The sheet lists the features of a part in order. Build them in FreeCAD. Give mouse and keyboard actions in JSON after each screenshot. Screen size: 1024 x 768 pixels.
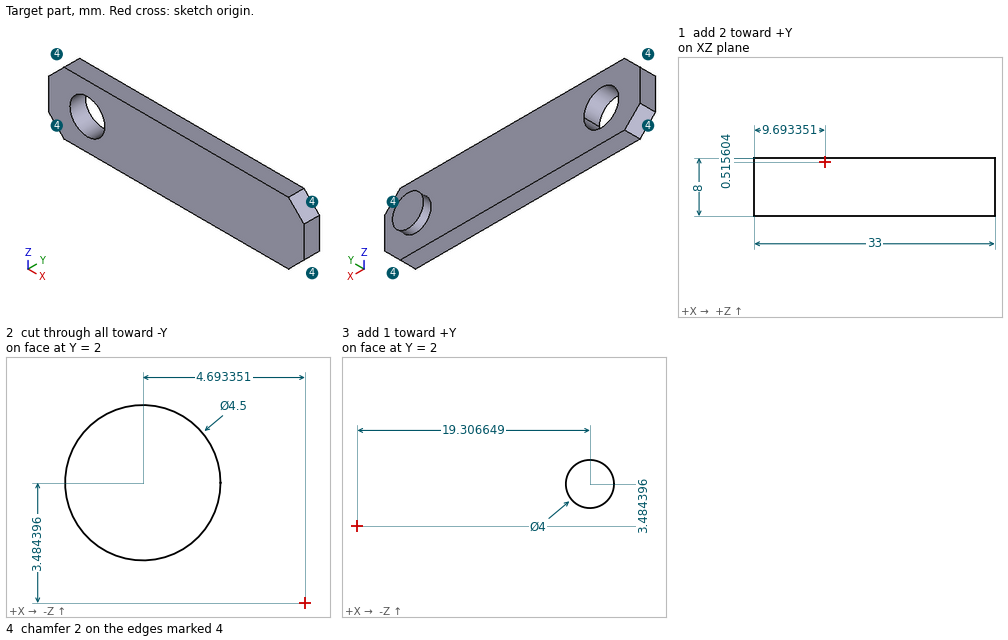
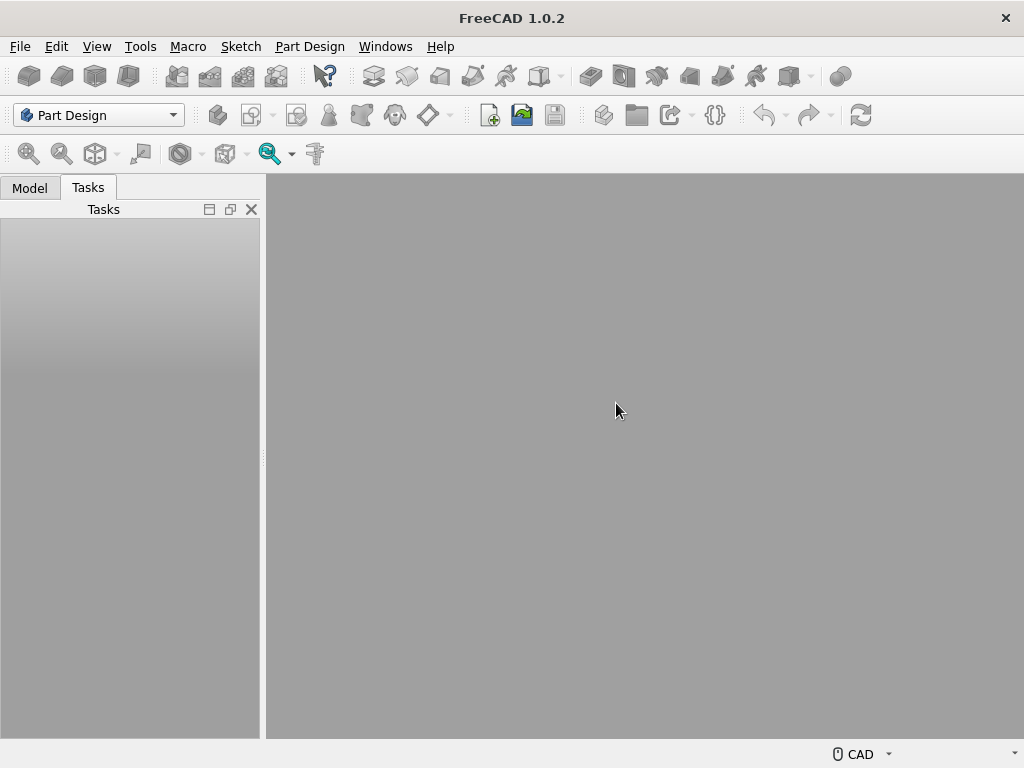
{"action": "key", "text": "ctrl+n"}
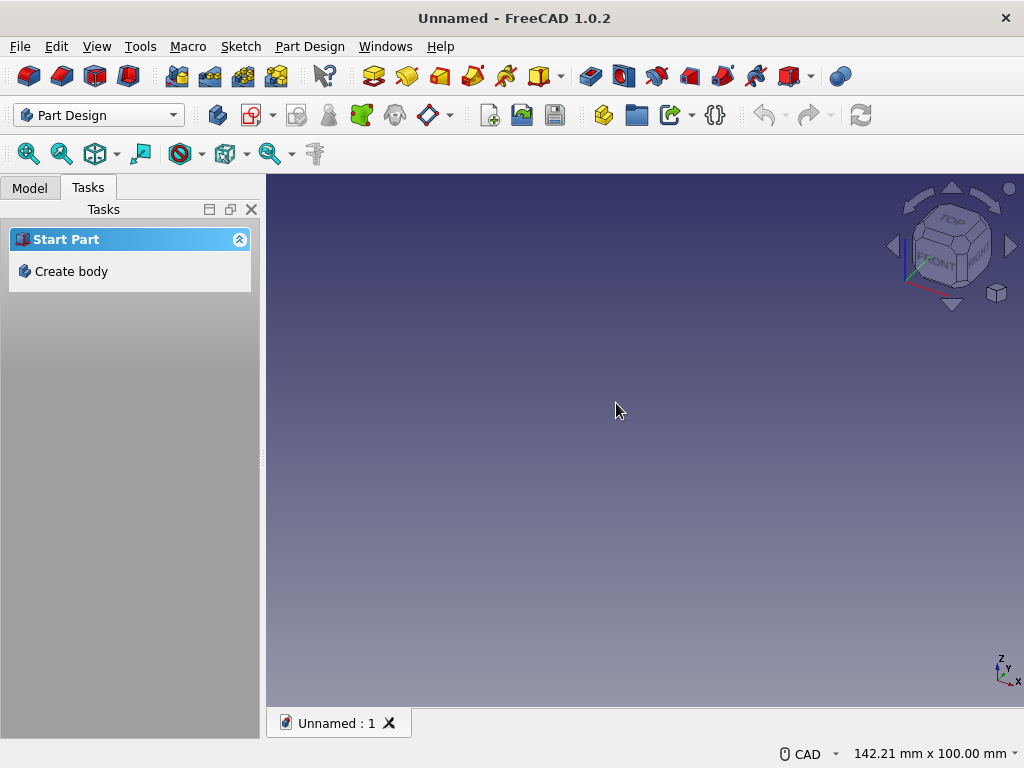
{"action": "left_click", "coordinate": [250, 116]}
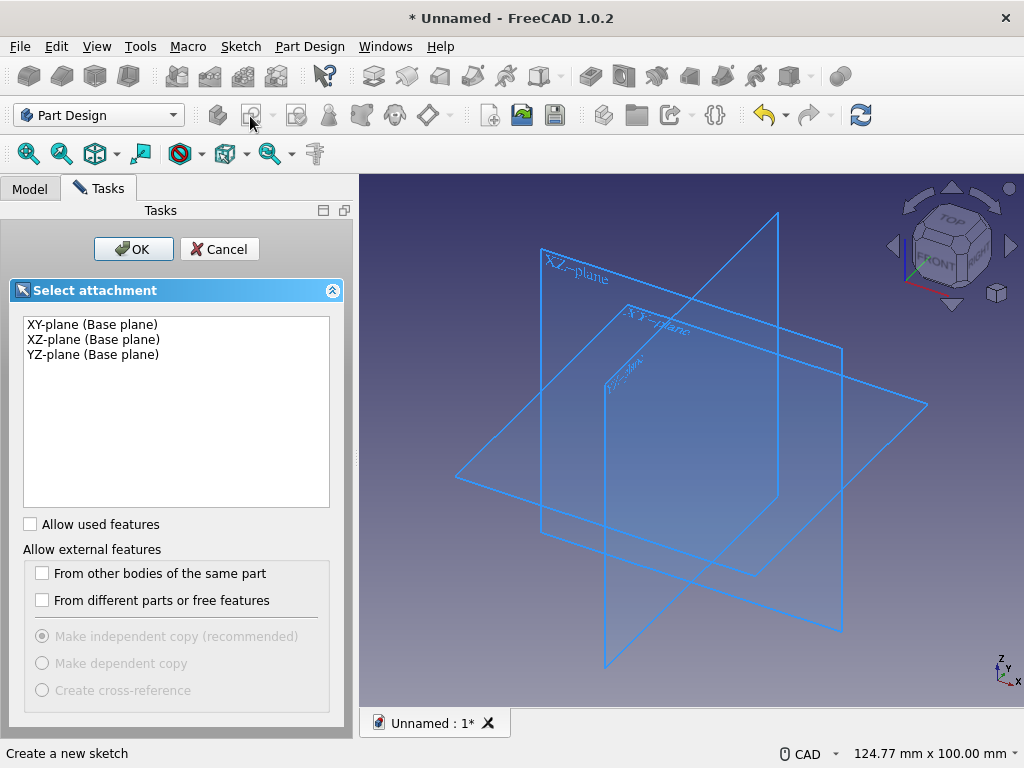
{"action": "left_click", "coordinate": [84, 340]}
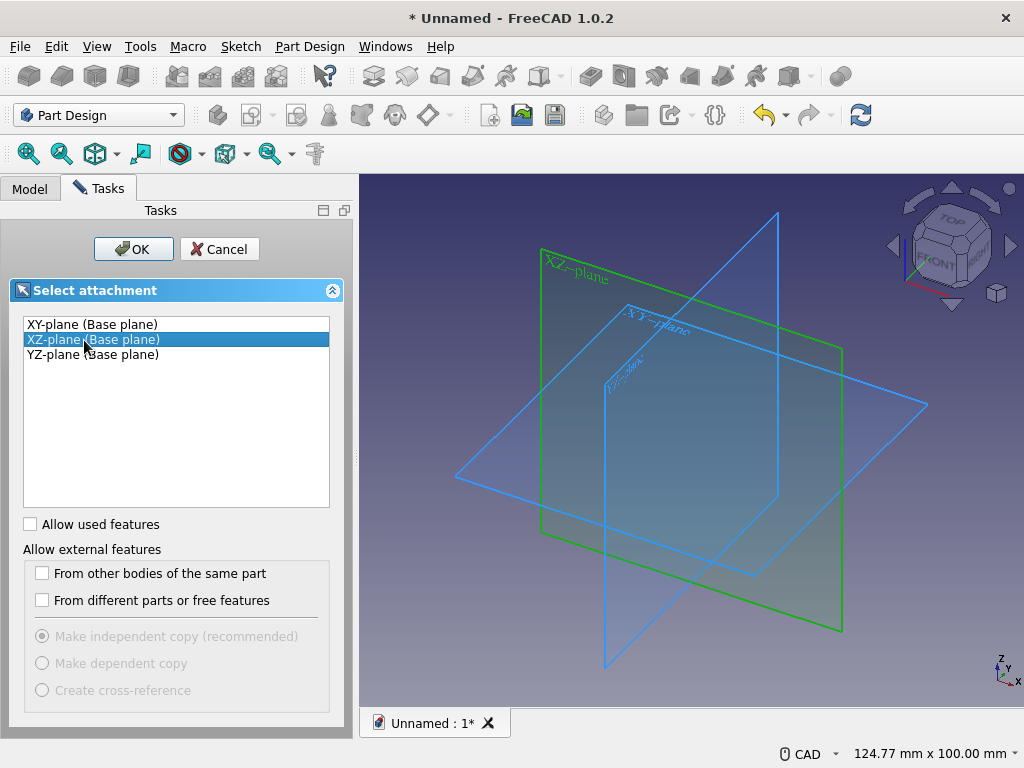
{"action": "left_click", "coordinate": [134, 249]}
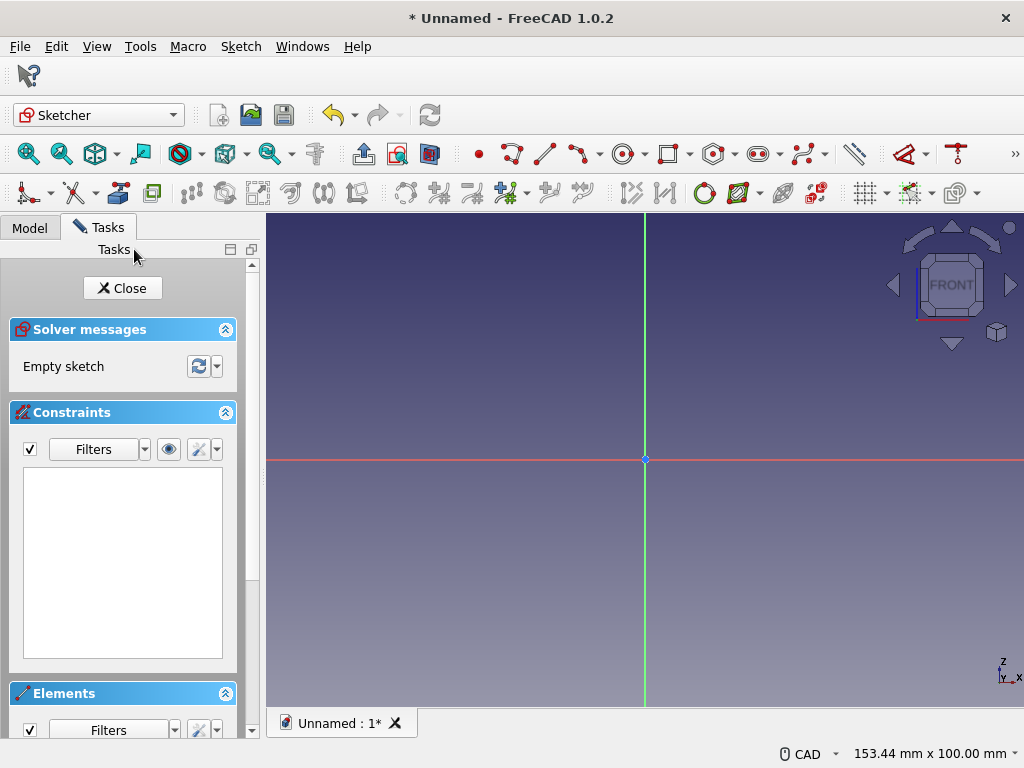
{"action": "scroll", "coordinate": [762, 491], "scroll_direction": "up", "scroll_amount": 4}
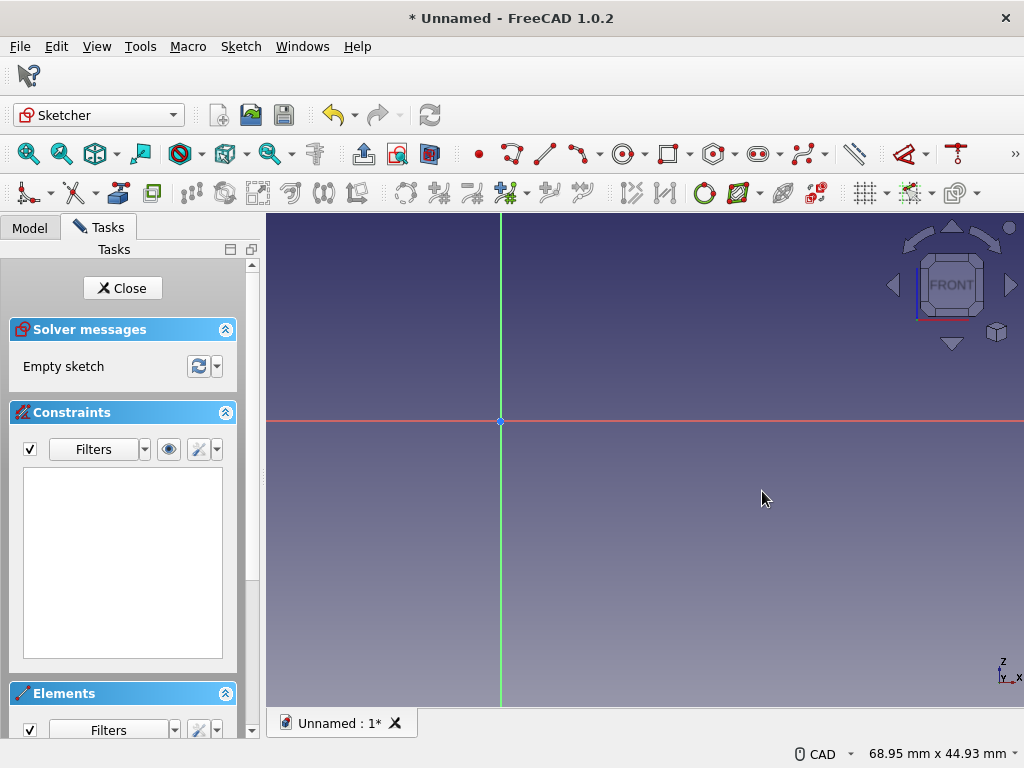
{"action": "left_click", "coordinate": [668, 154]}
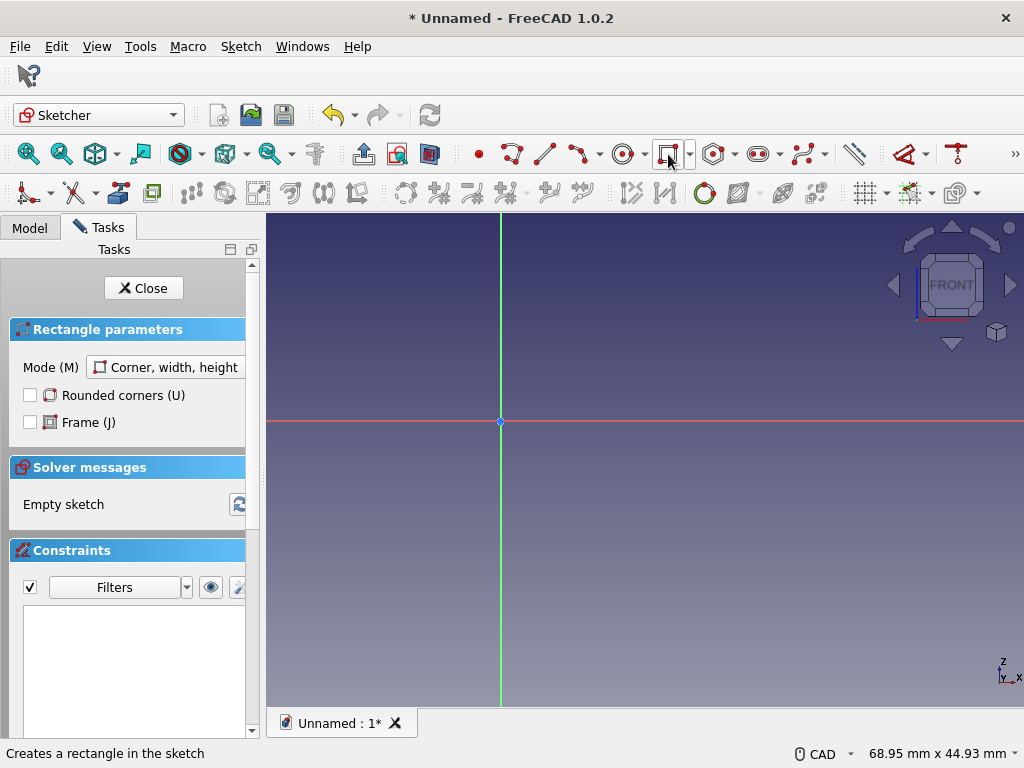
{"action": "scroll", "coordinate": [394, 416], "scroll_direction": "up", "scroll_amount": 6}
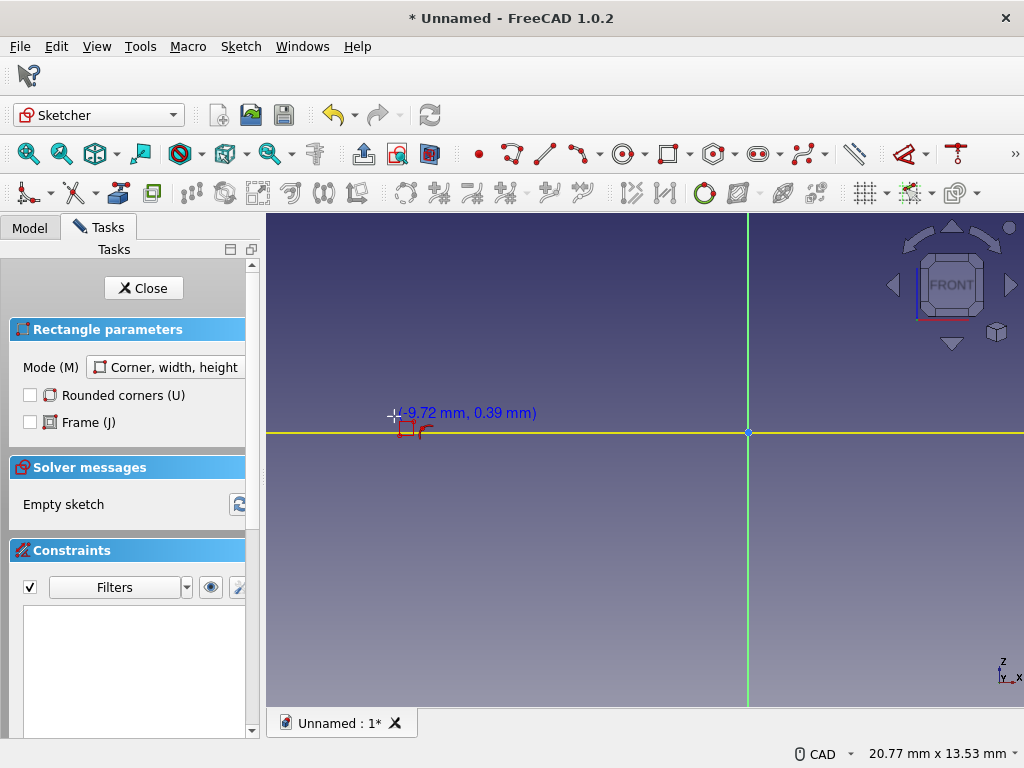
{"action": "left_click", "coordinate": [394, 414]}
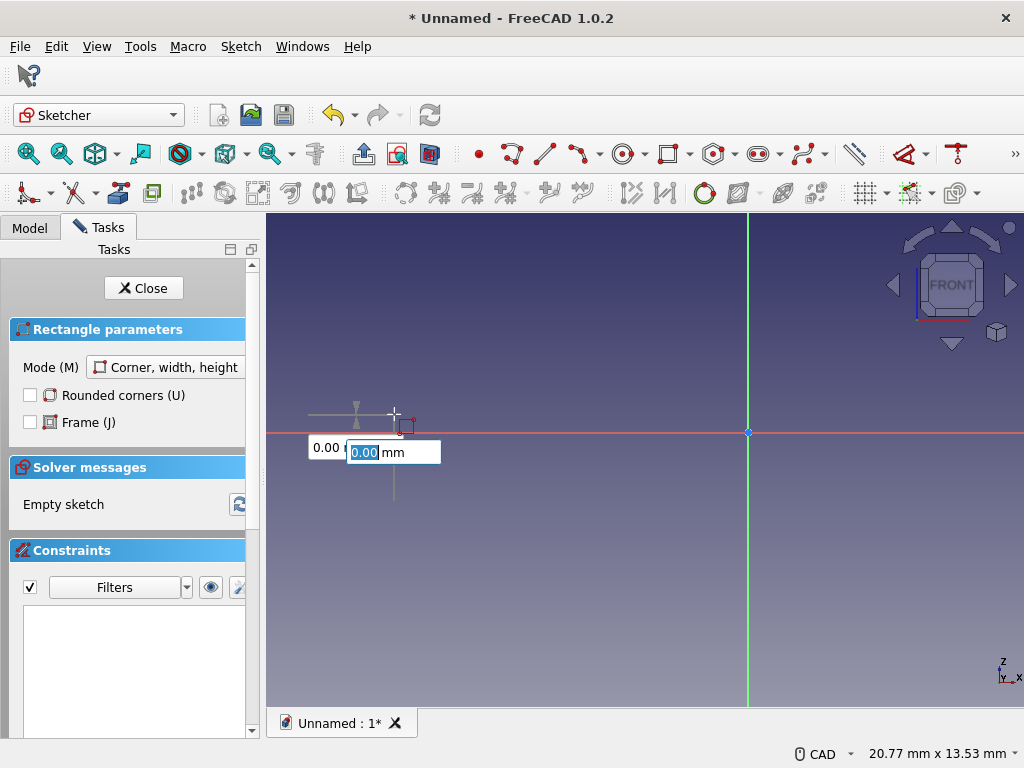
{"action": "scroll", "coordinate": [395, 417], "scroll_direction": "down", "scroll_amount": 6}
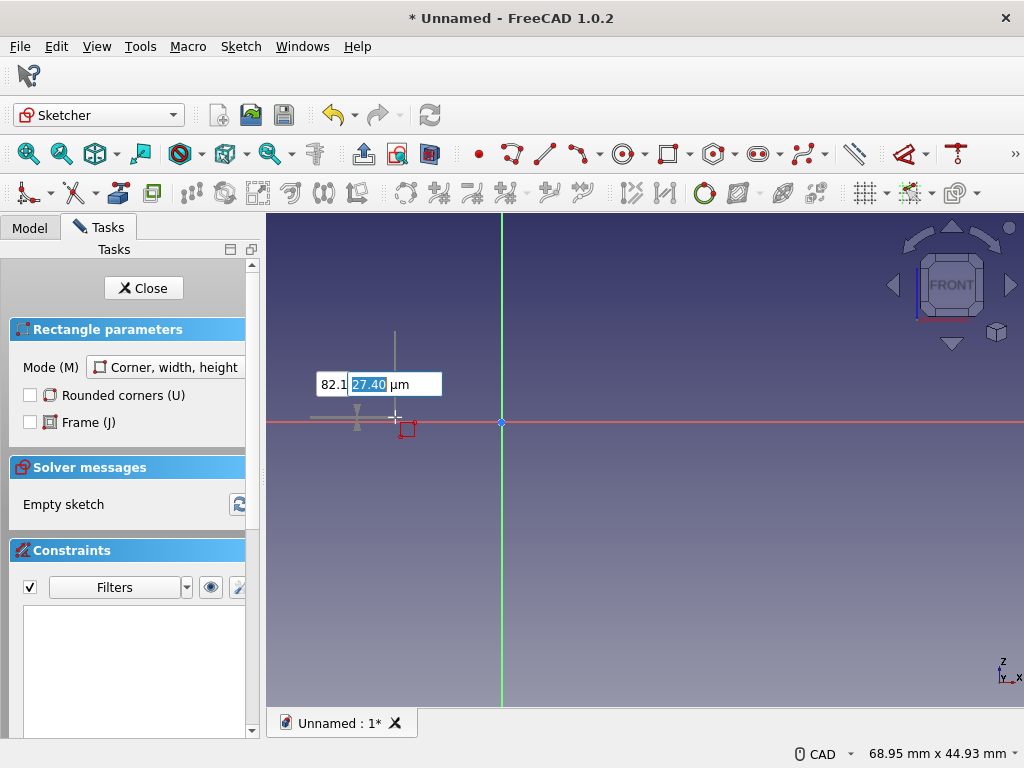
{"action": "left_click", "coordinate": [758, 504]}
{"action": "key", "text": "Escape"}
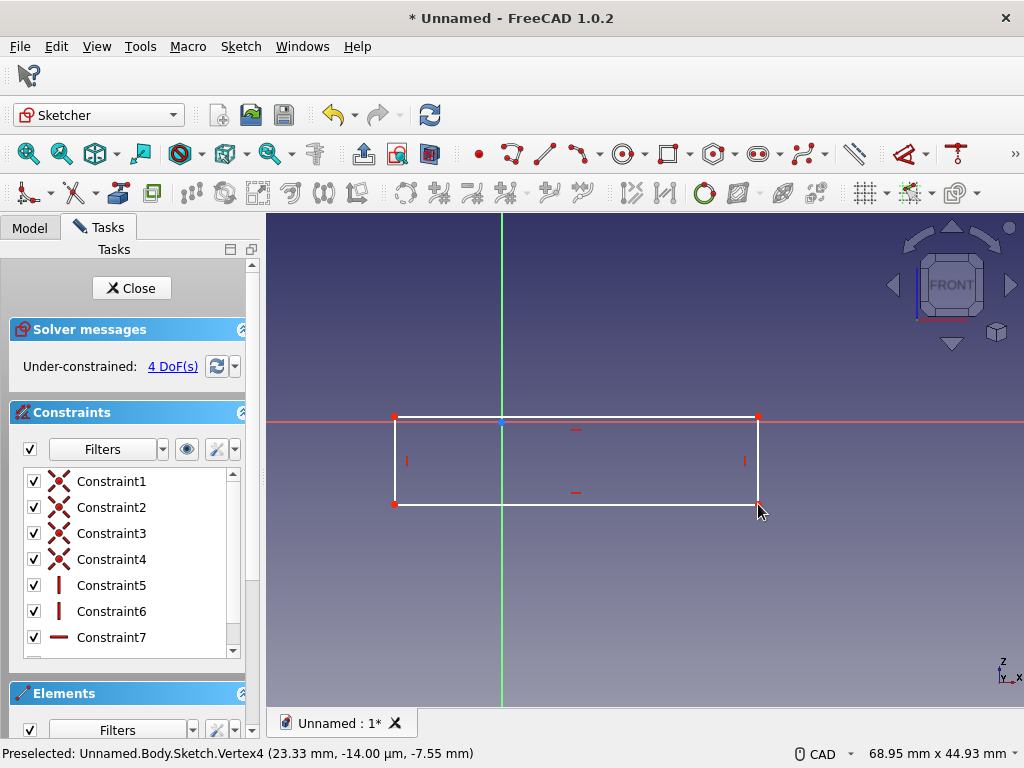
{"action": "left_click", "coordinate": [904, 154]}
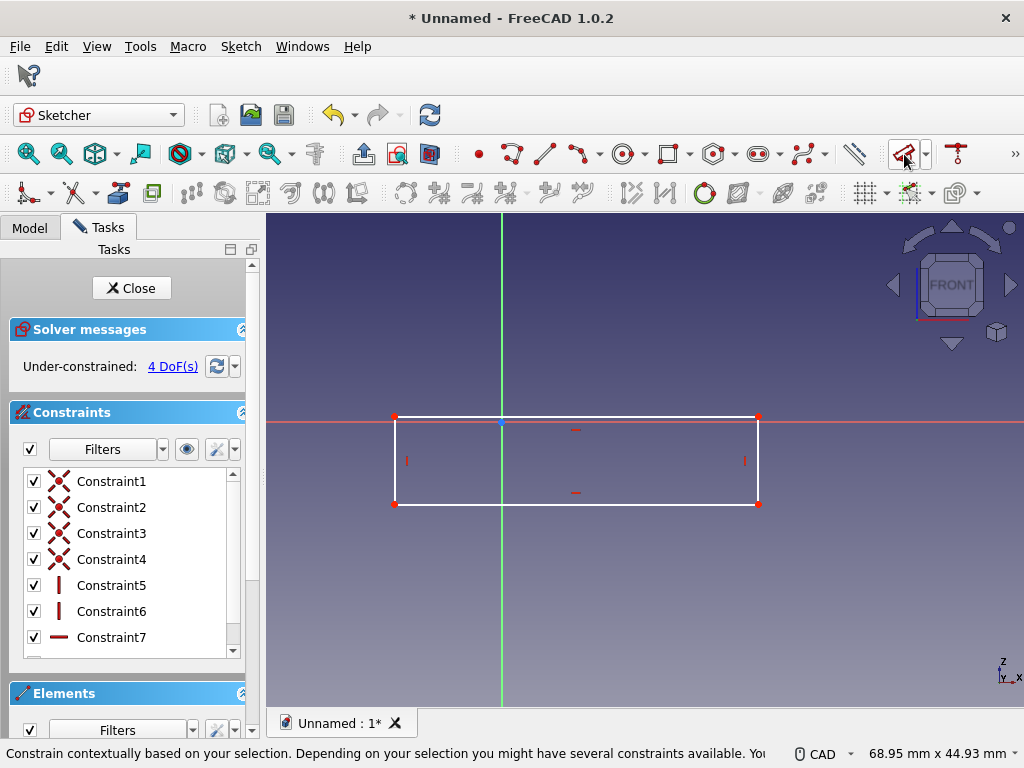
{"action": "left_click", "coordinate": [395, 443]}
{"action": "left_click", "coordinate": [361, 461]}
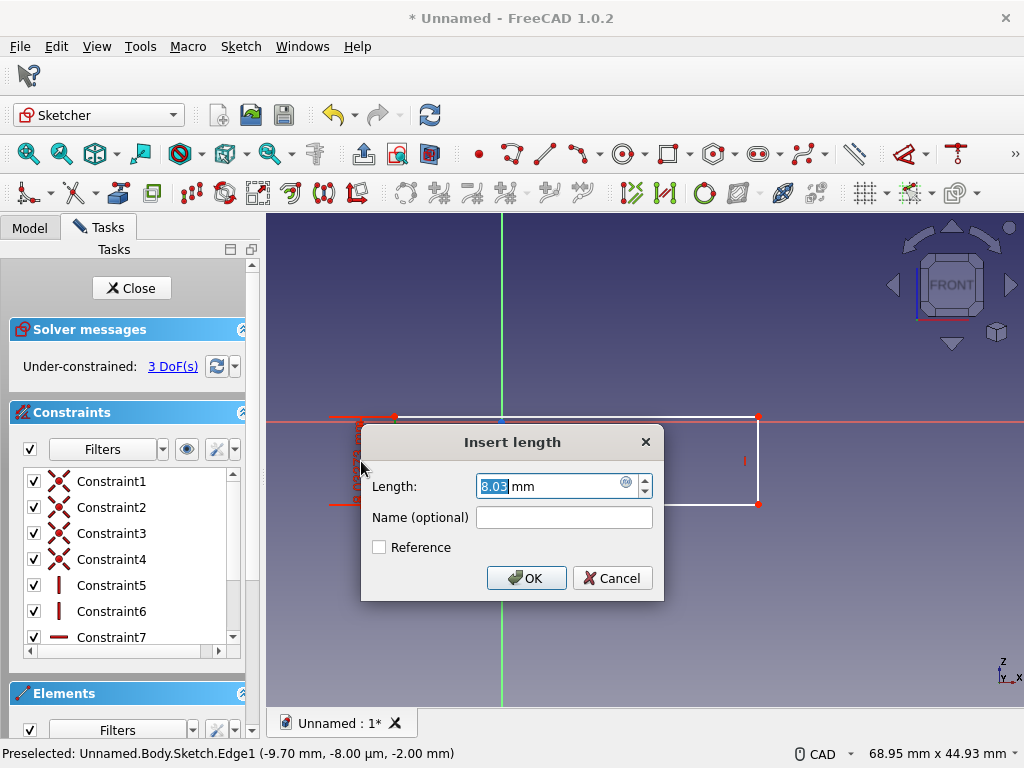
{"action": "type", "text": "8"}
{"action": "key", "text": "Return"}